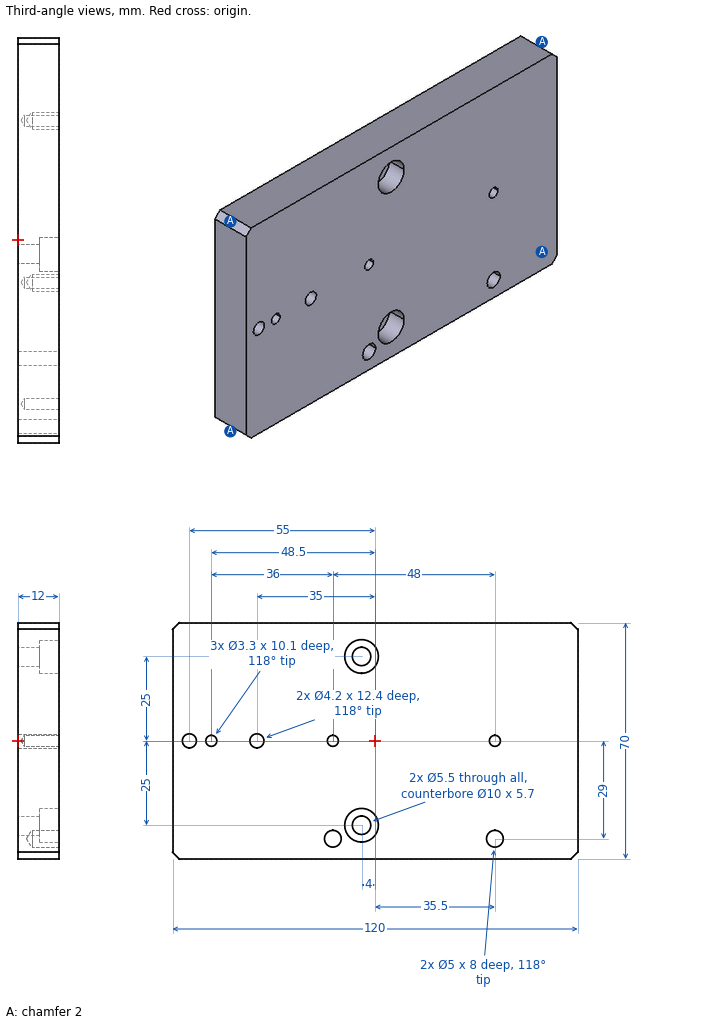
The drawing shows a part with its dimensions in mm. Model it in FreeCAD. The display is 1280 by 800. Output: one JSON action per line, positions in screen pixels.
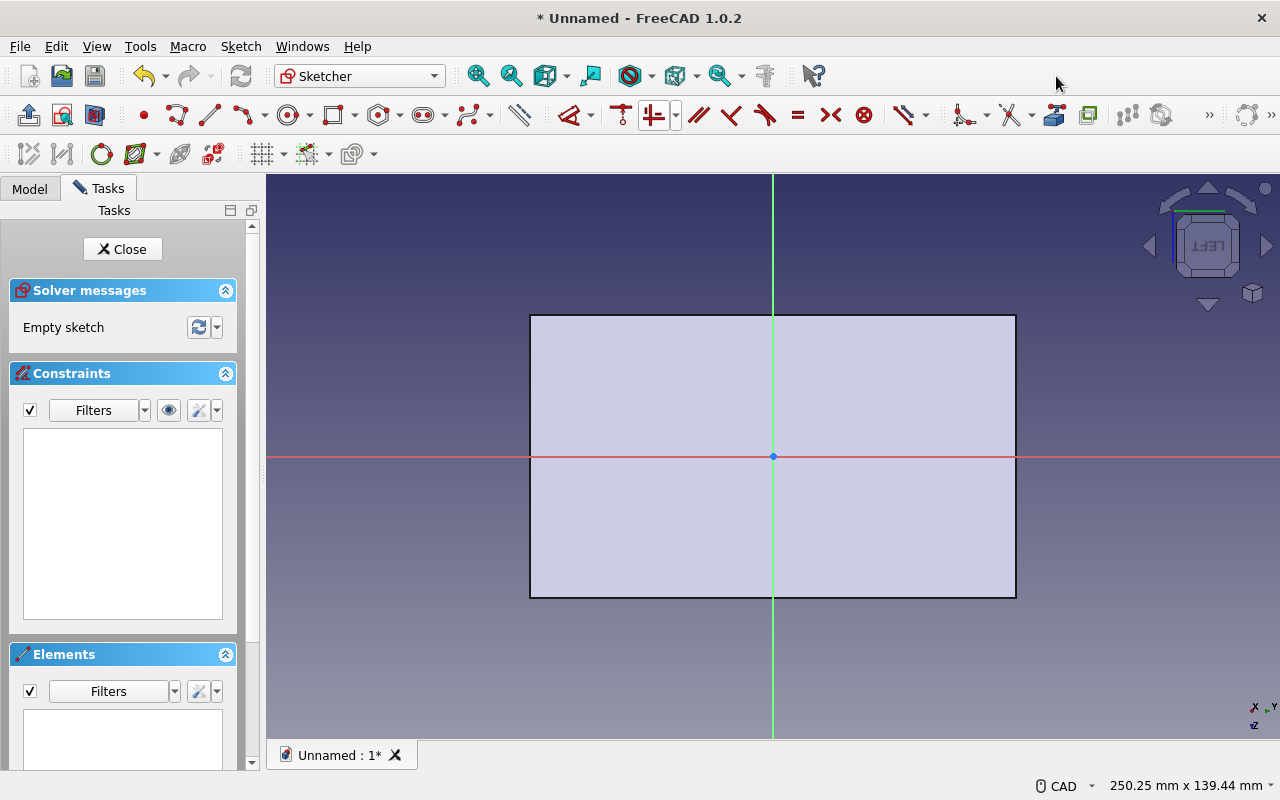
{"action": "scroll", "coordinate": [630, 456], "scroll_direction": "up", "scroll_amount": 5}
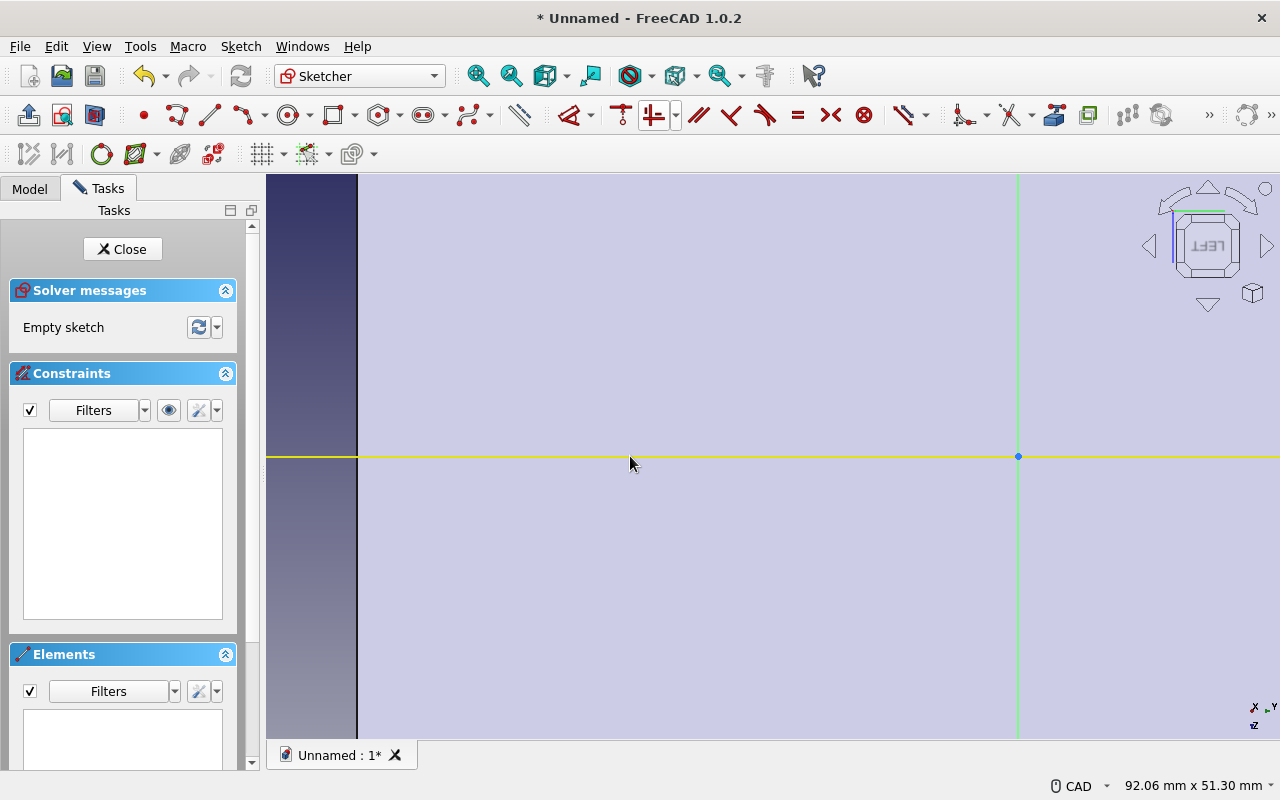
{"action": "left_click", "coordinate": [288, 116]}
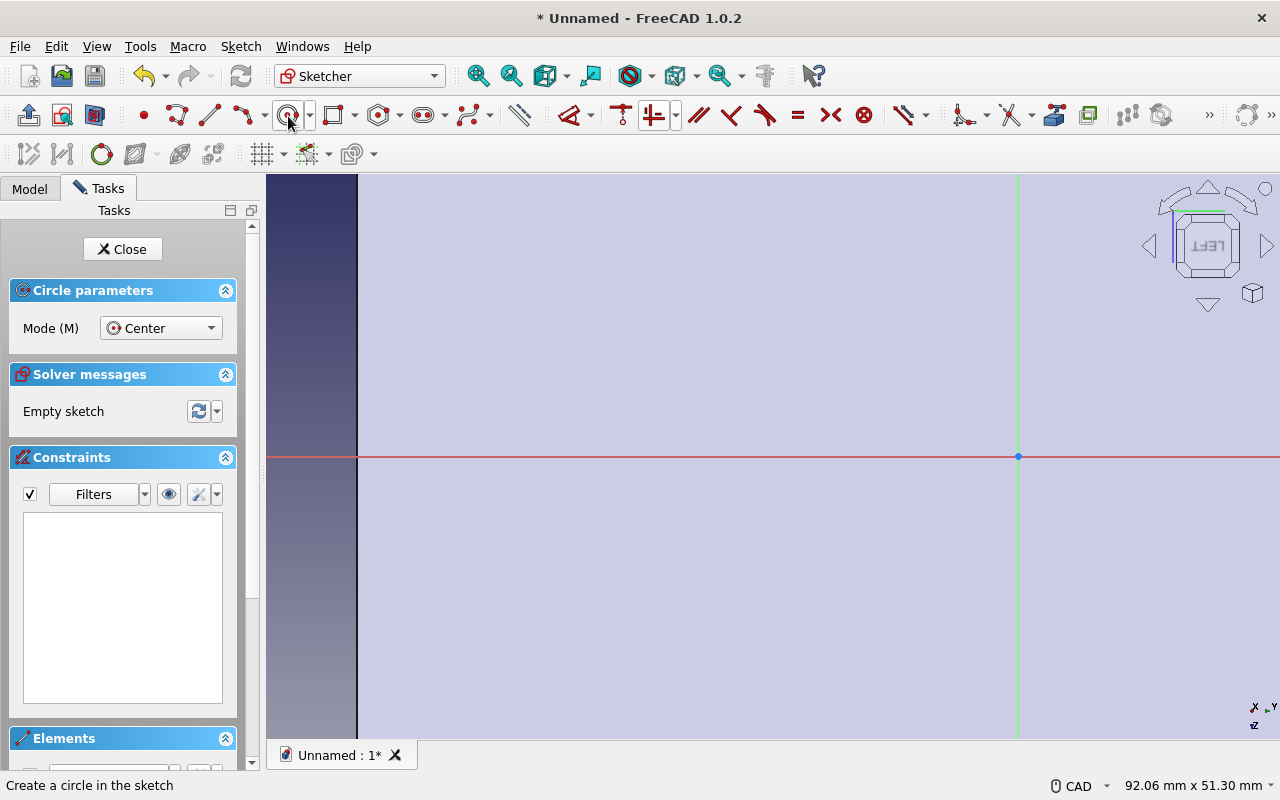
{"action": "left_click", "coordinate": [633, 456]}
{"action": "left_click", "coordinate": [649, 440]}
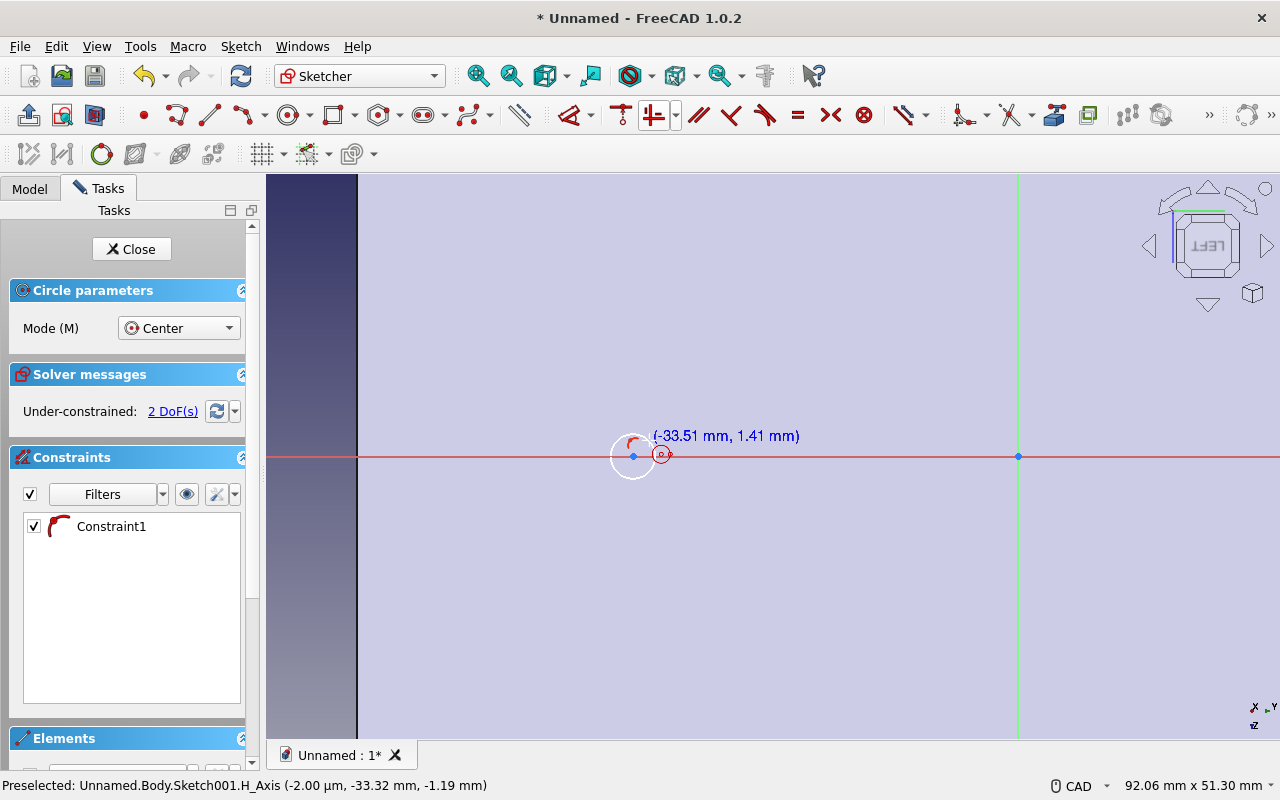
{"action": "left_click", "coordinate": [412, 456]}
{"action": "left_click", "coordinate": [429, 440]}
{"action": "key", "text": "Escape"}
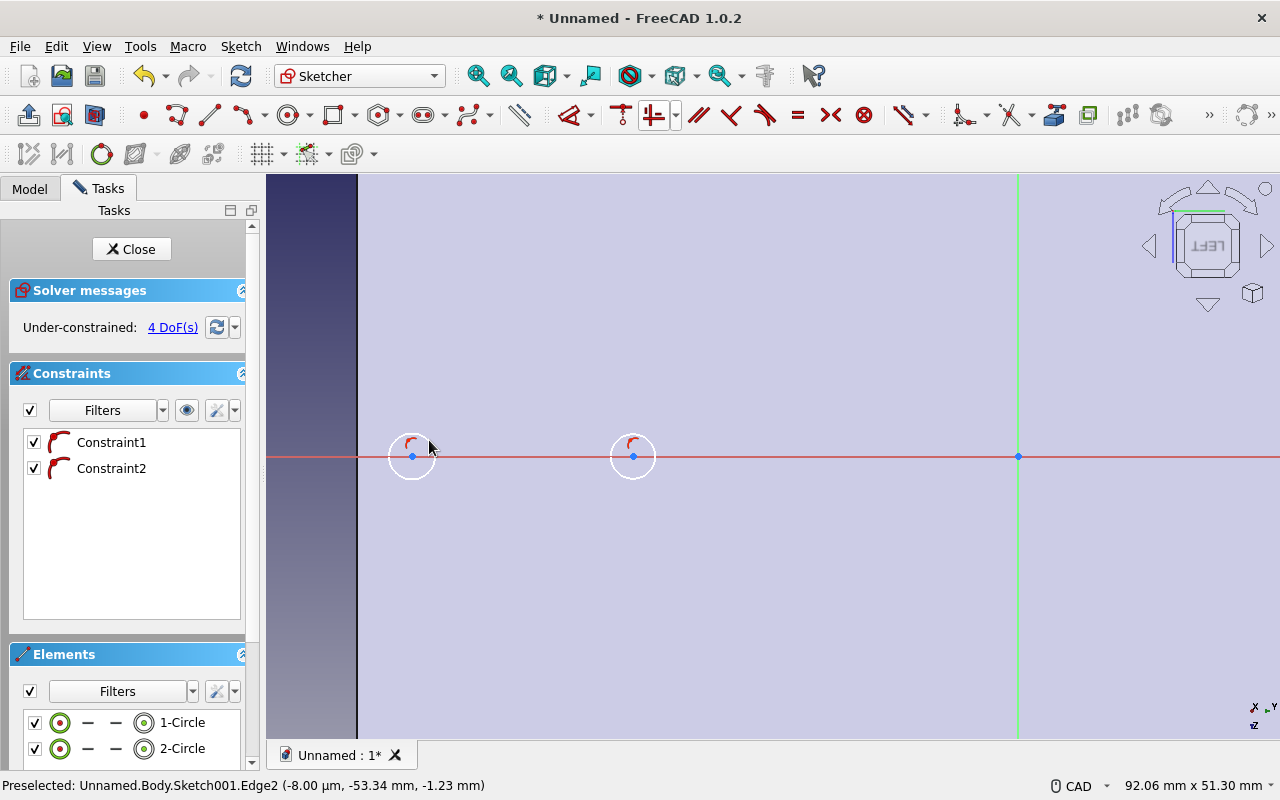
{"action": "left_click", "coordinate": [649, 441]}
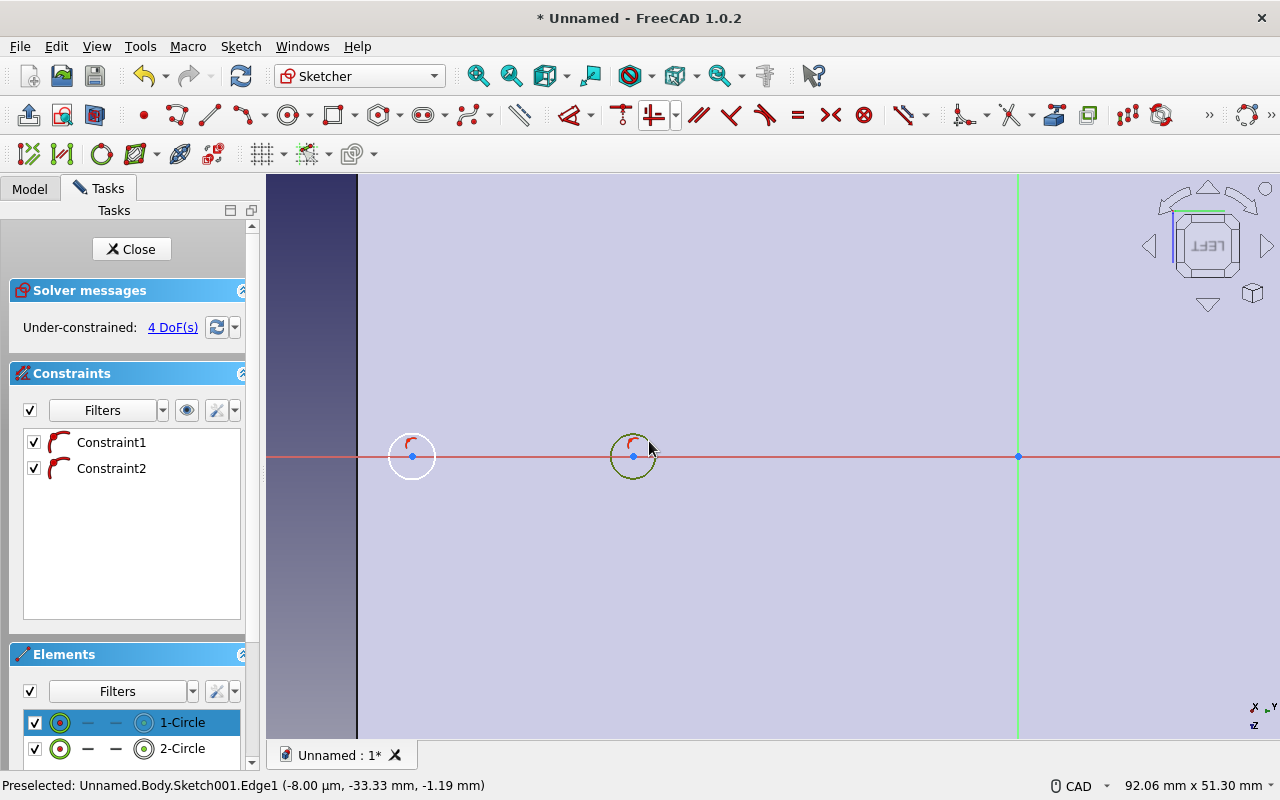
{"action": "left_click", "coordinate": [428, 440]}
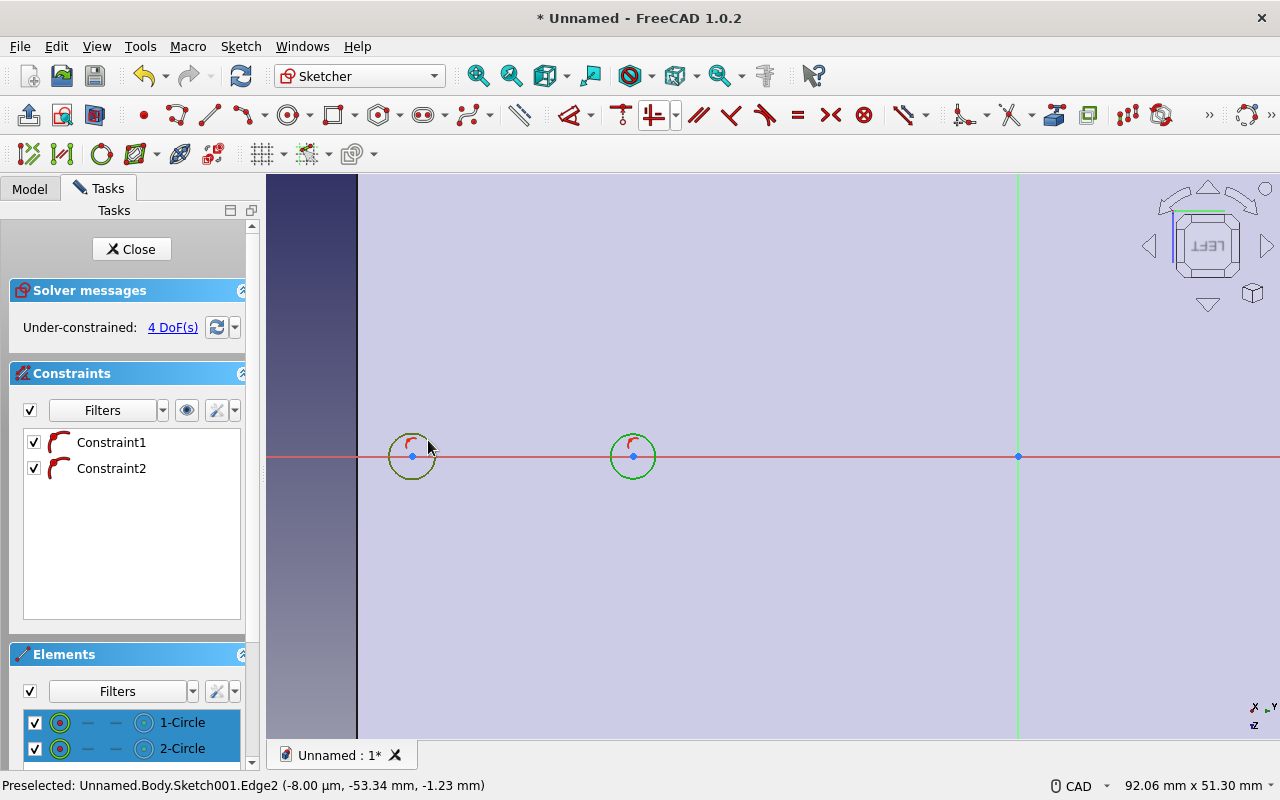
{"action": "left_click", "coordinate": [798, 116]}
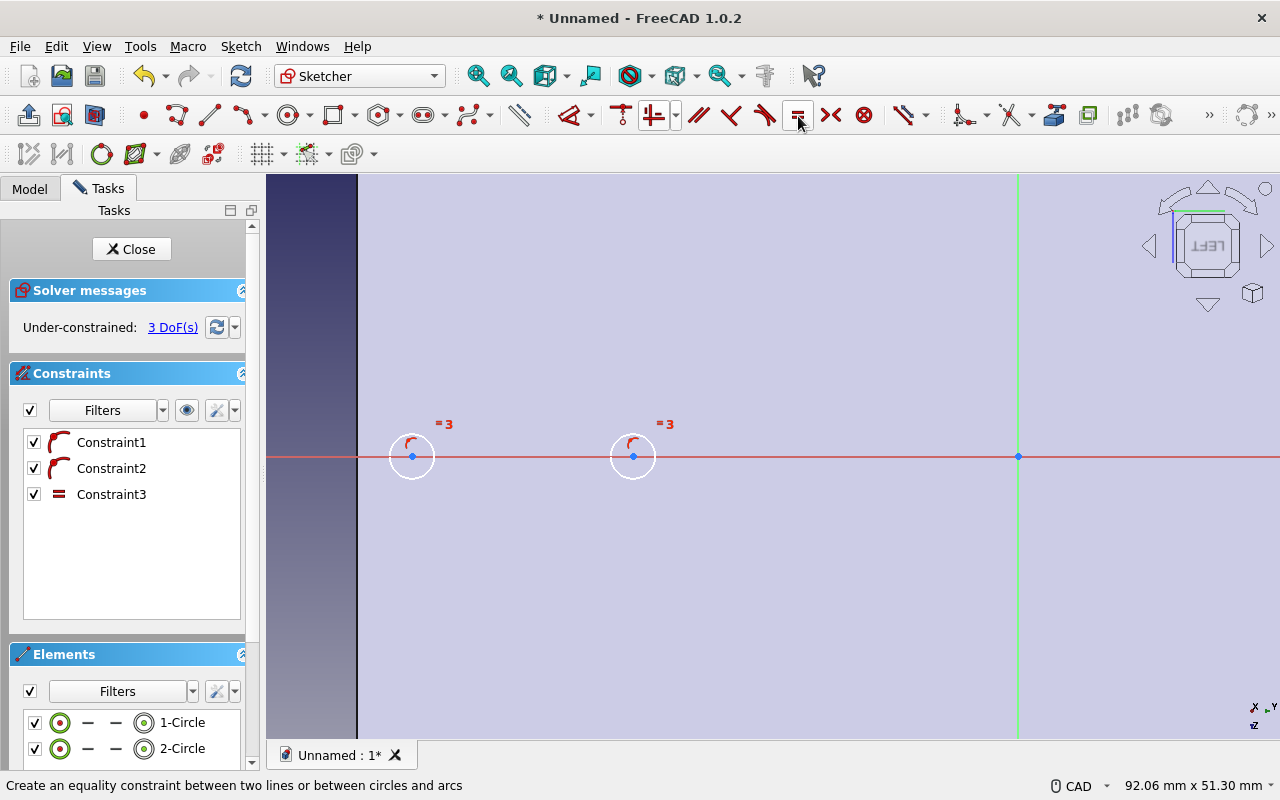
{"action": "left_click", "coordinate": [568, 116]}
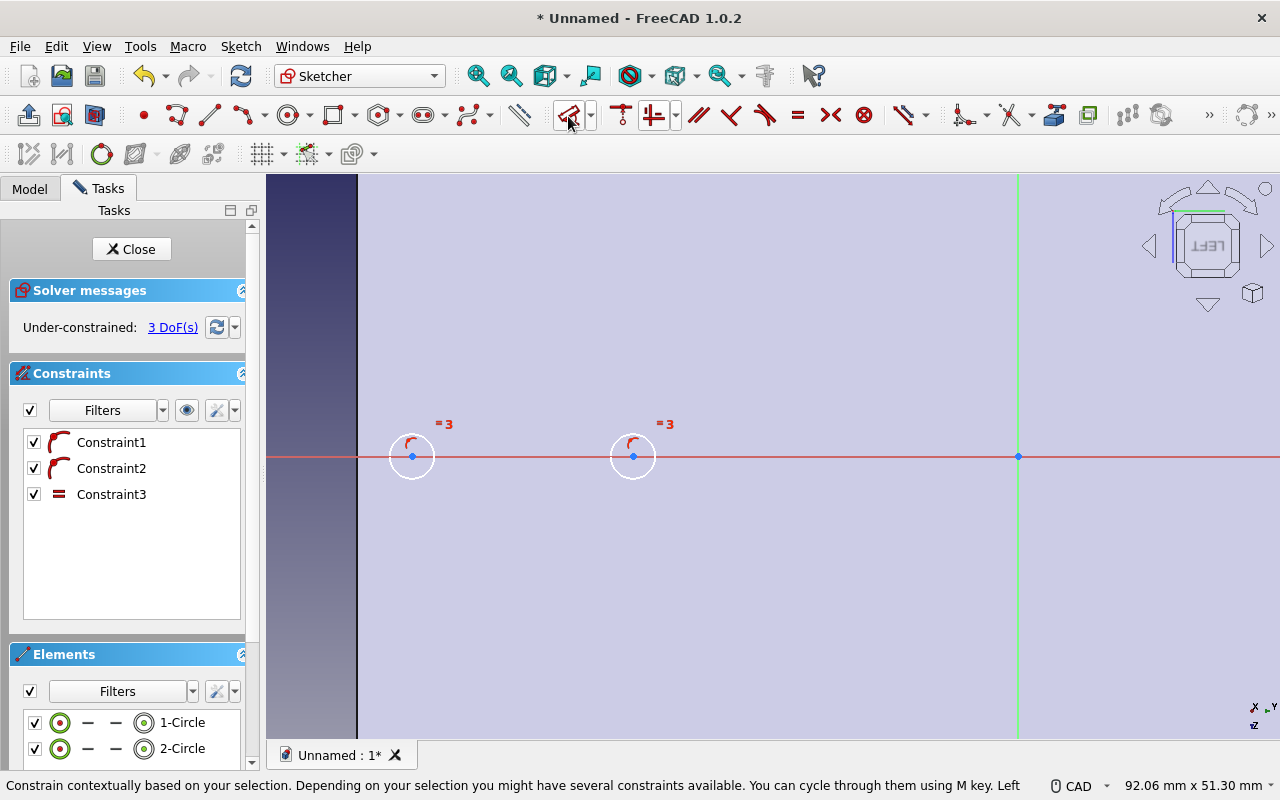
{"action": "left_click", "coordinate": [649, 441]}
{"action": "left_click", "coordinate": [672, 419]}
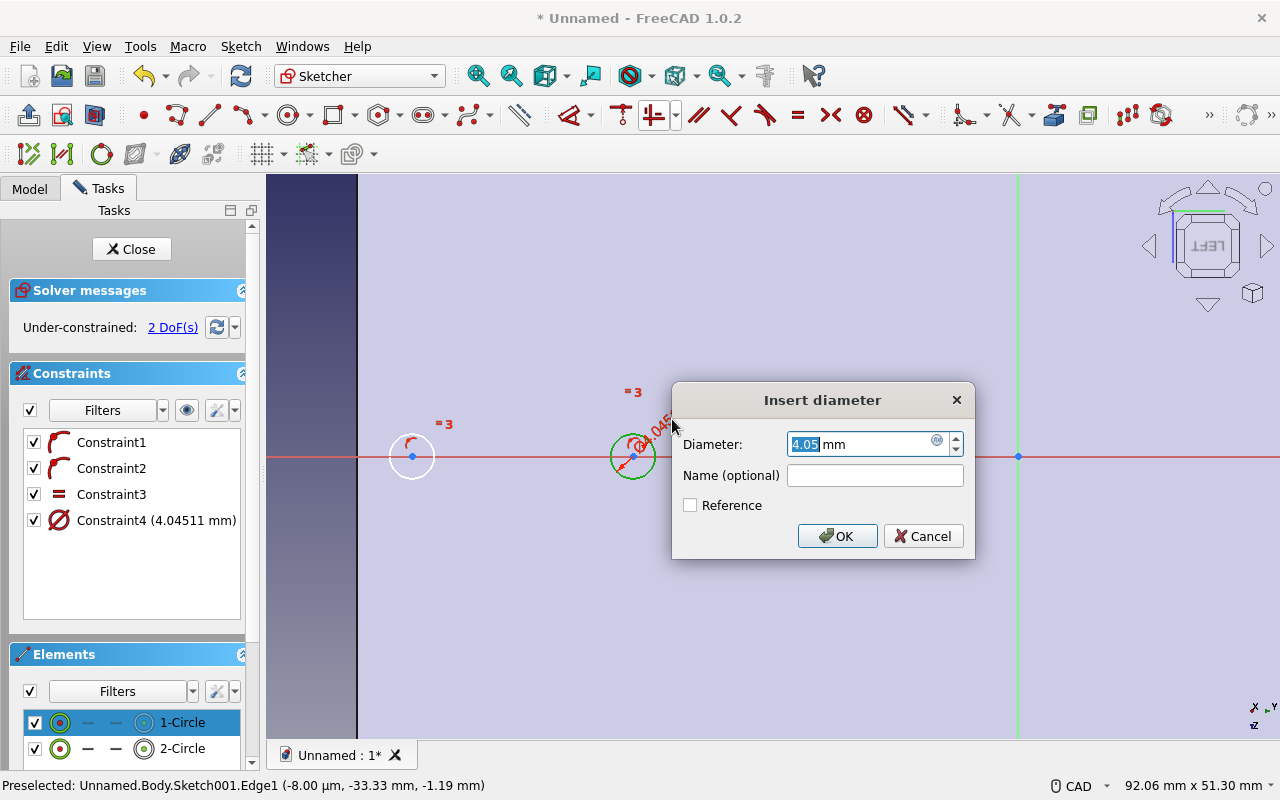
{"action": "type", "text": "4.2"}
{"action": "key", "text": "Return"}